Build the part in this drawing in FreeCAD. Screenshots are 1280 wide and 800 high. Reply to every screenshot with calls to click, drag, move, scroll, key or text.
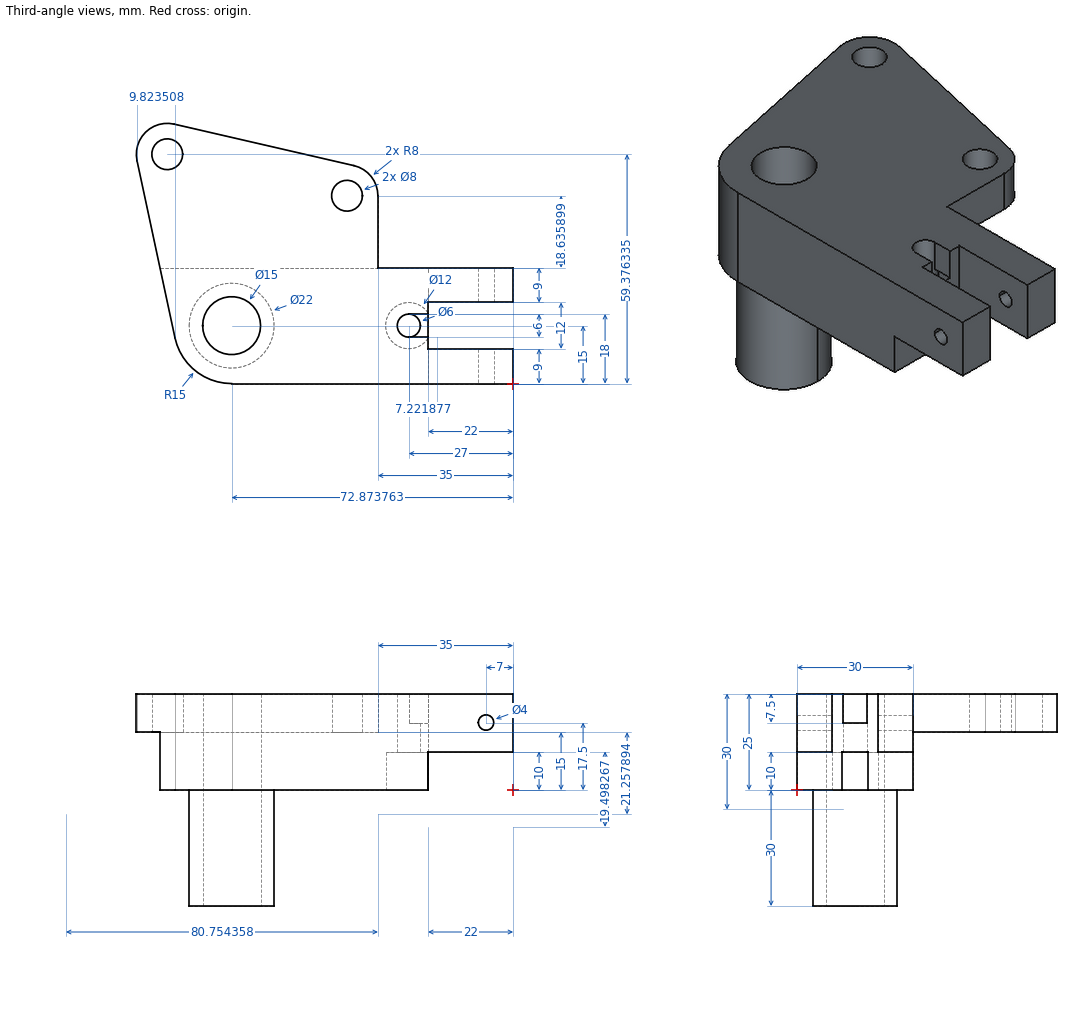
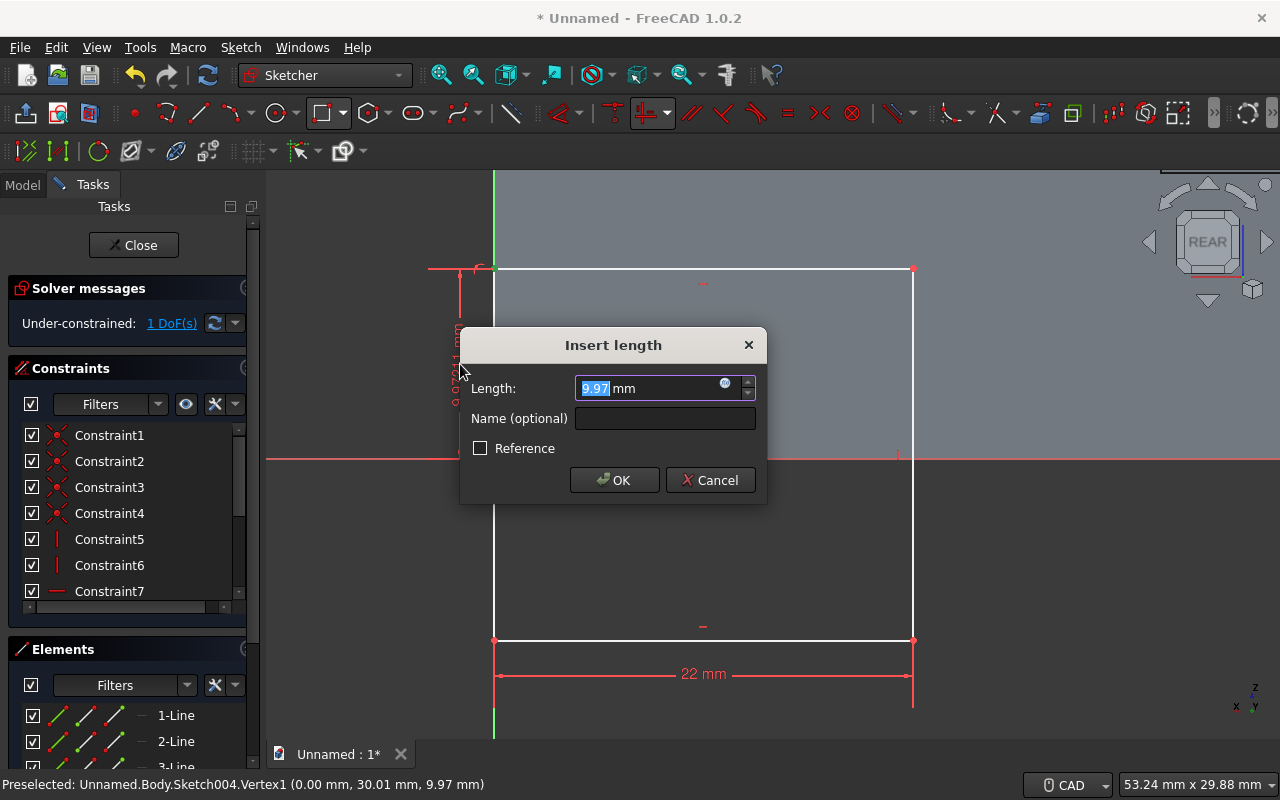
text(10)
key(Return)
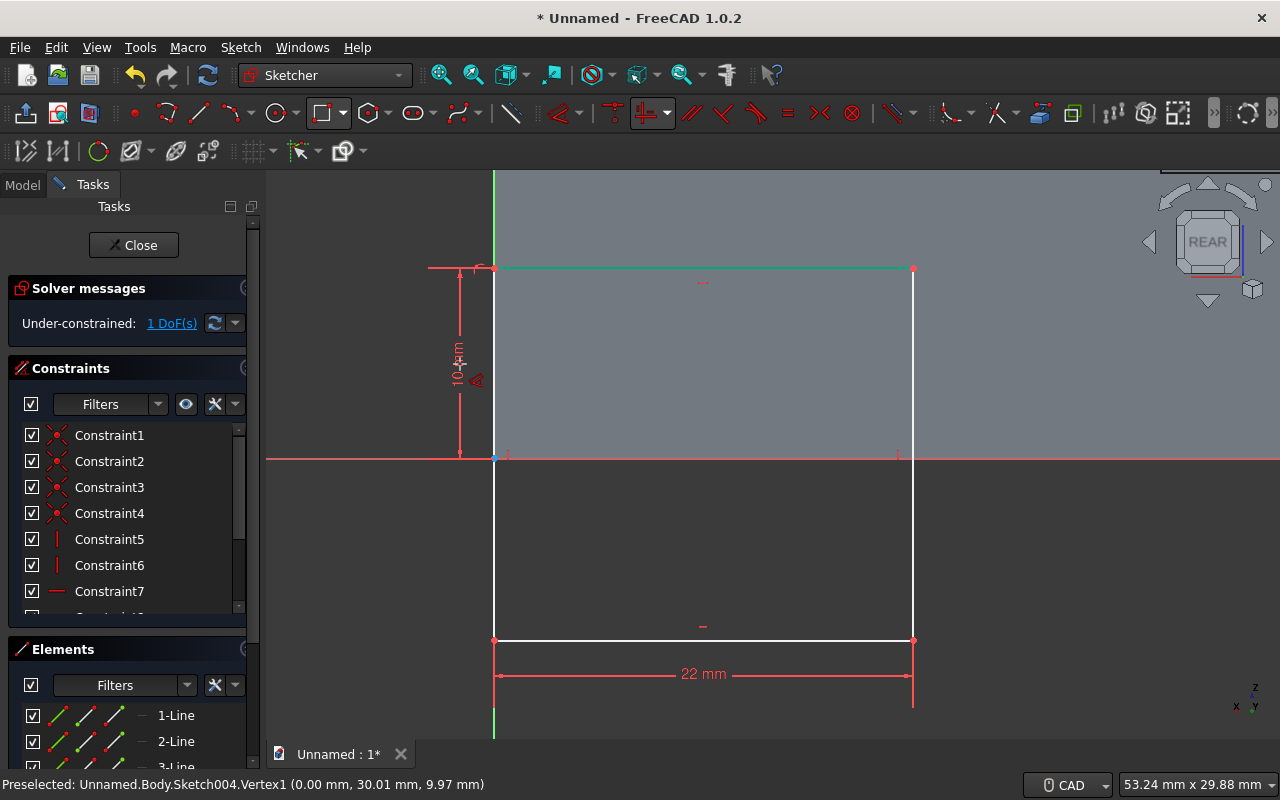
click(494, 380)
click(460, 540)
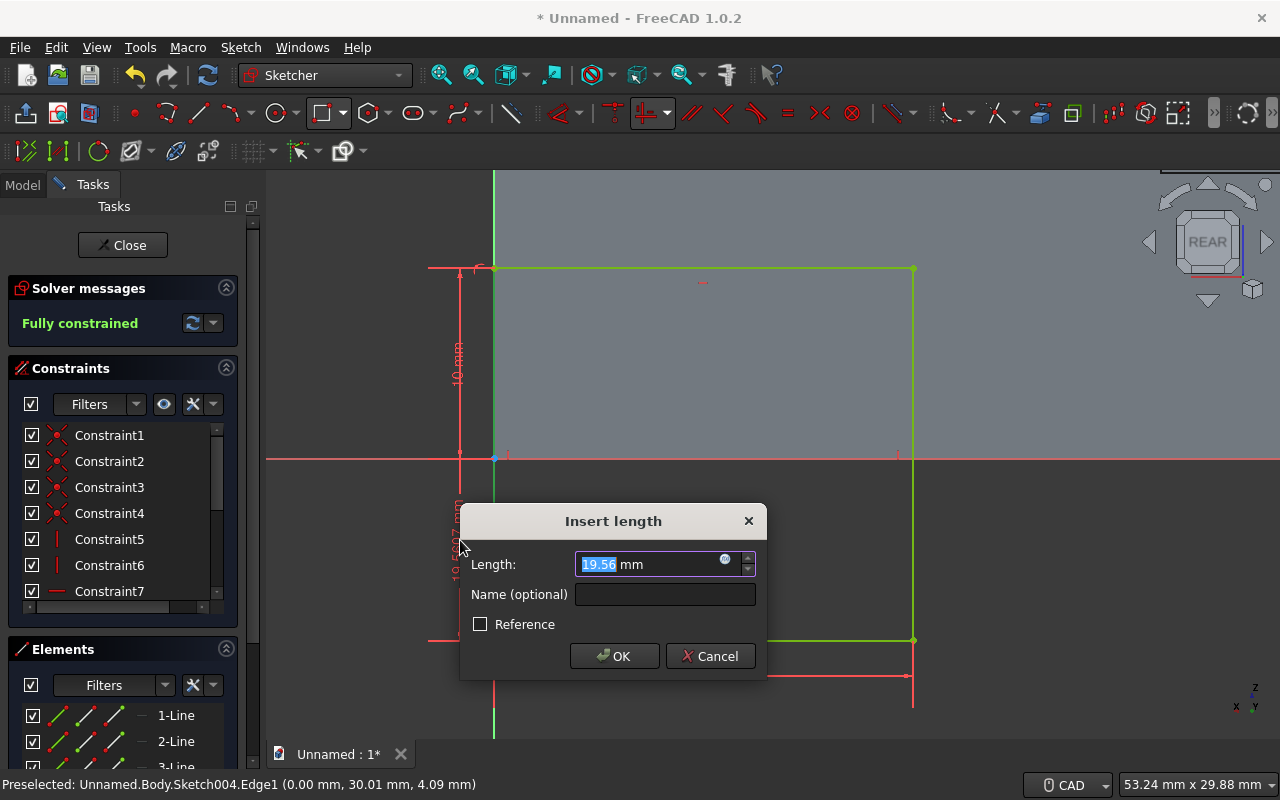
text(19.498267)
key(Return)
key(Escape)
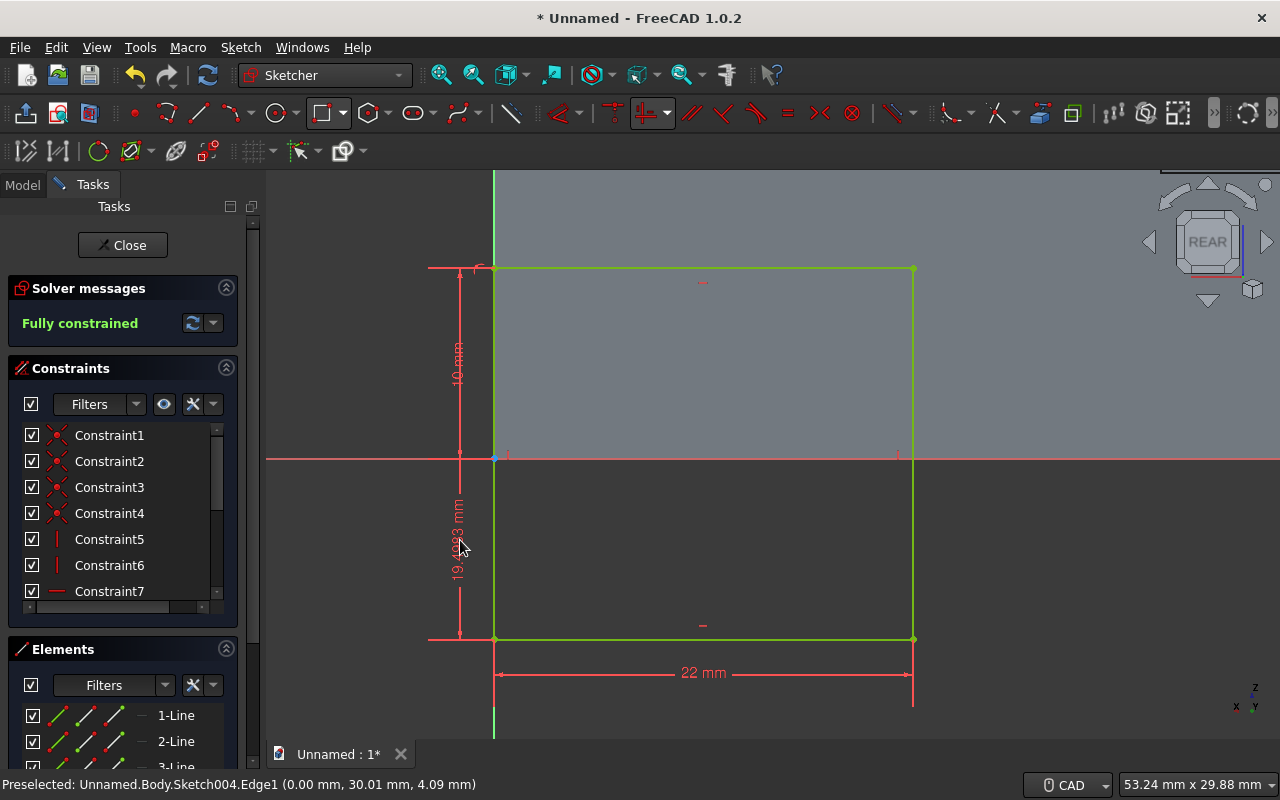
click(123, 245)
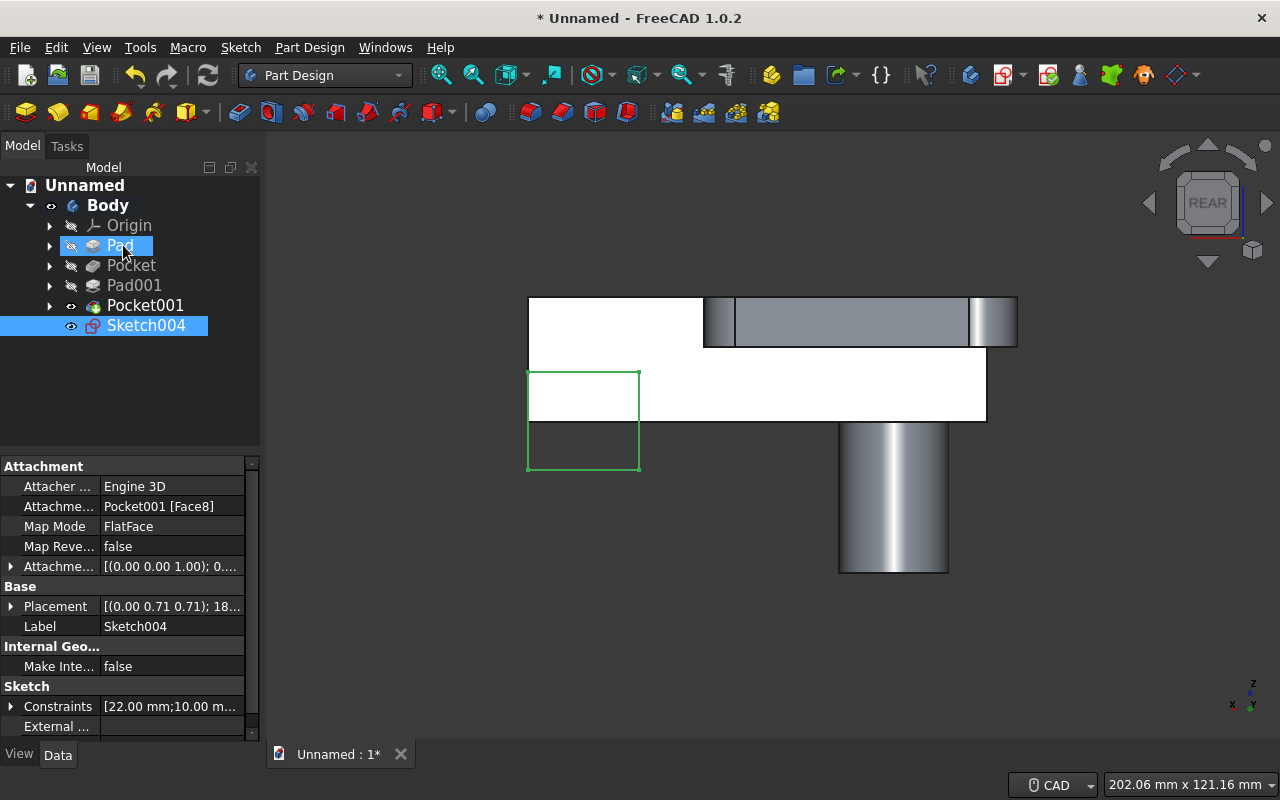
click(240, 112)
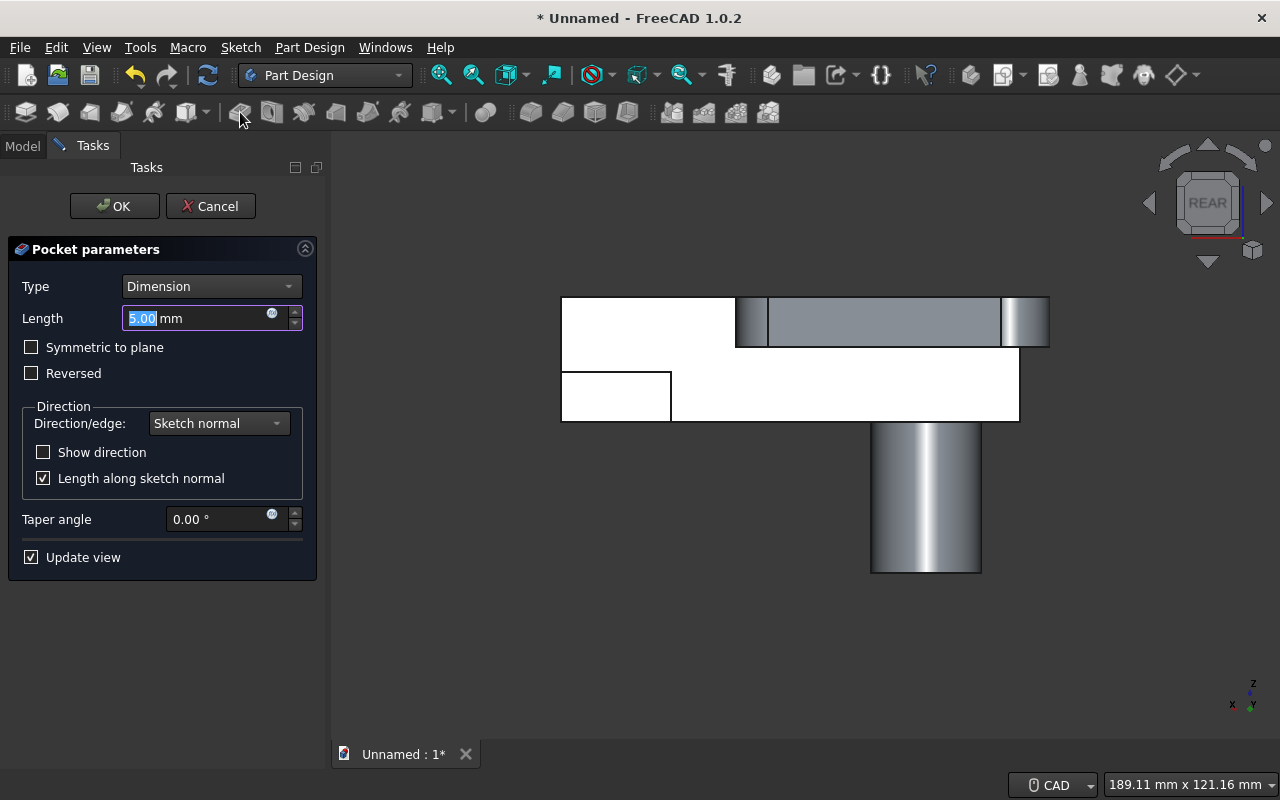
click(212, 286)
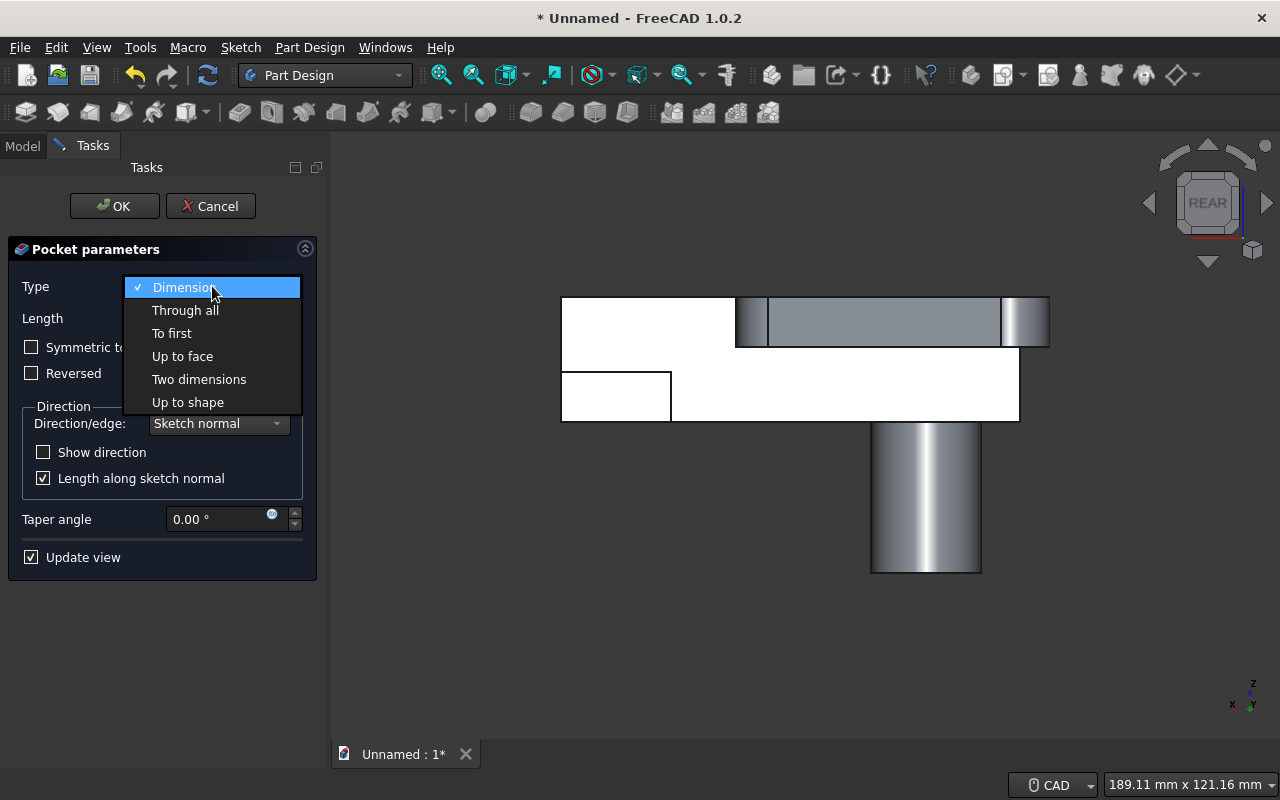
click(212, 310)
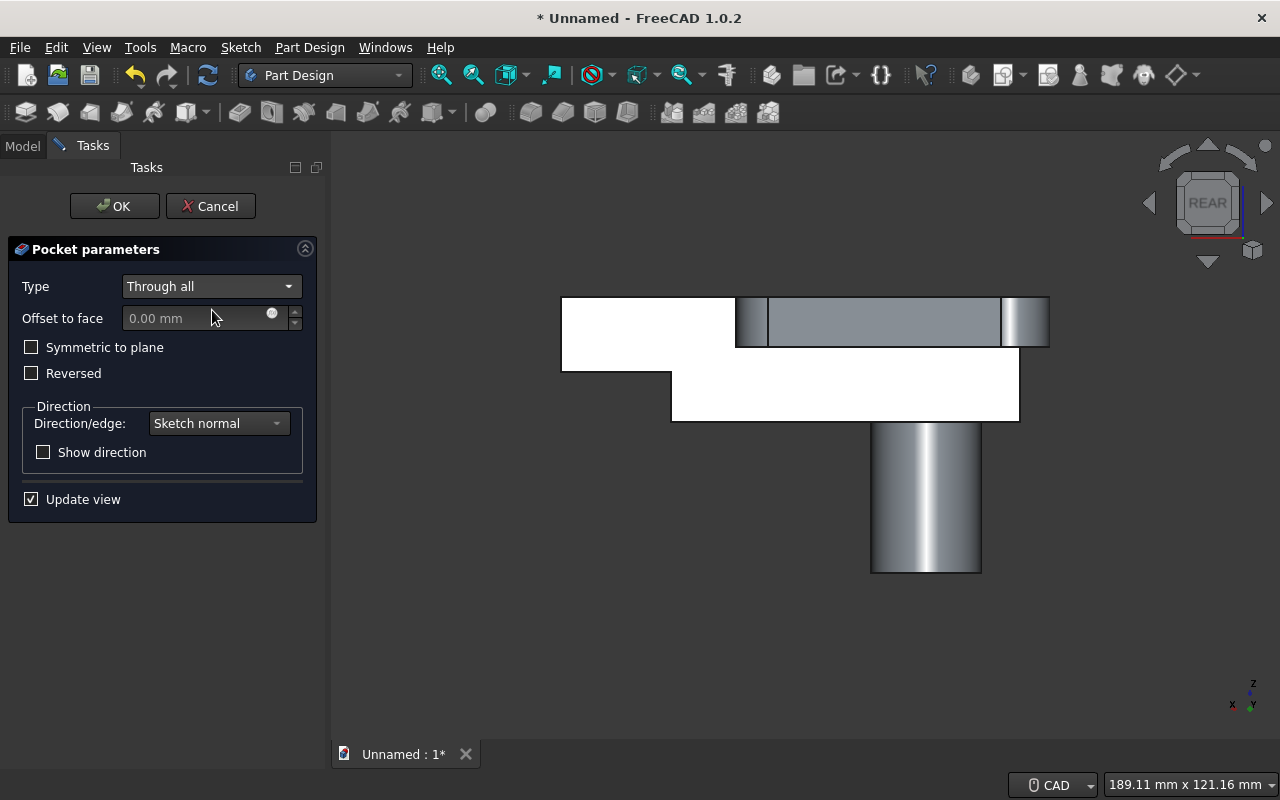
click(115, 206)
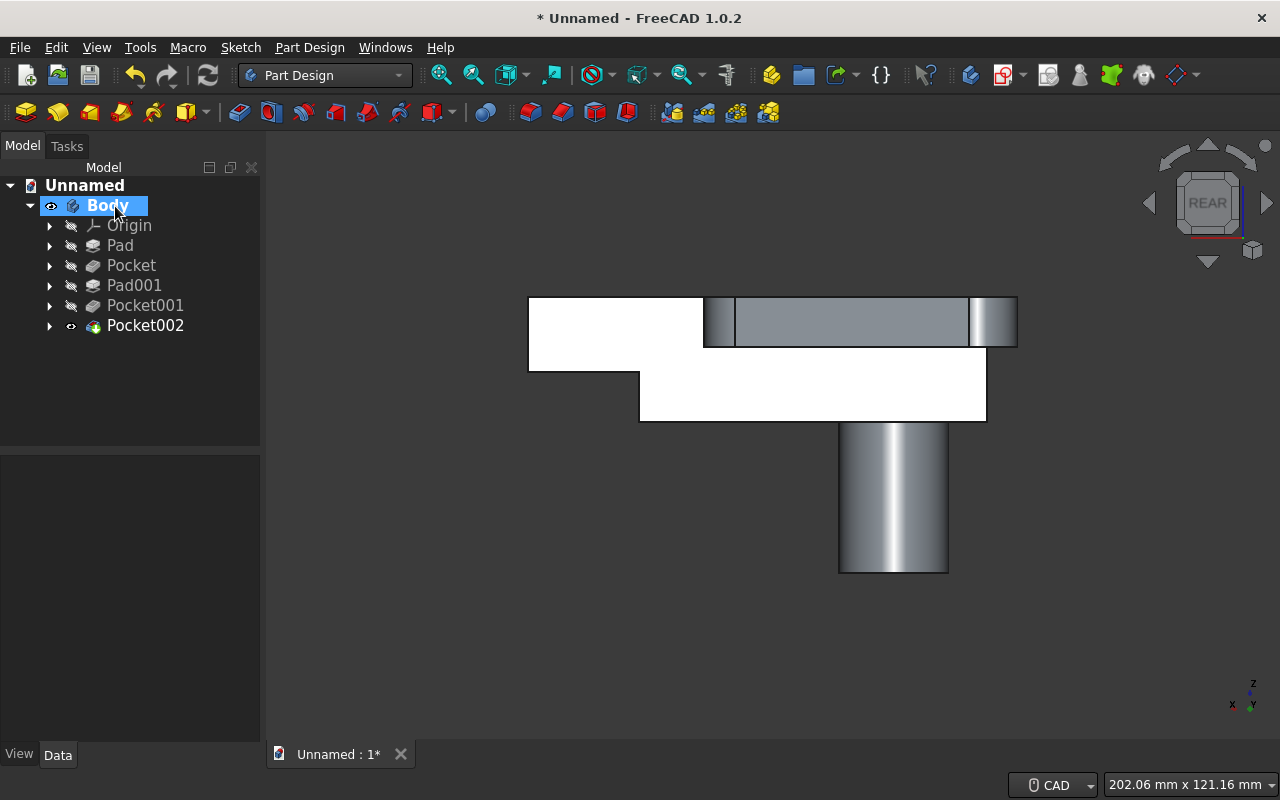
click(692, 377)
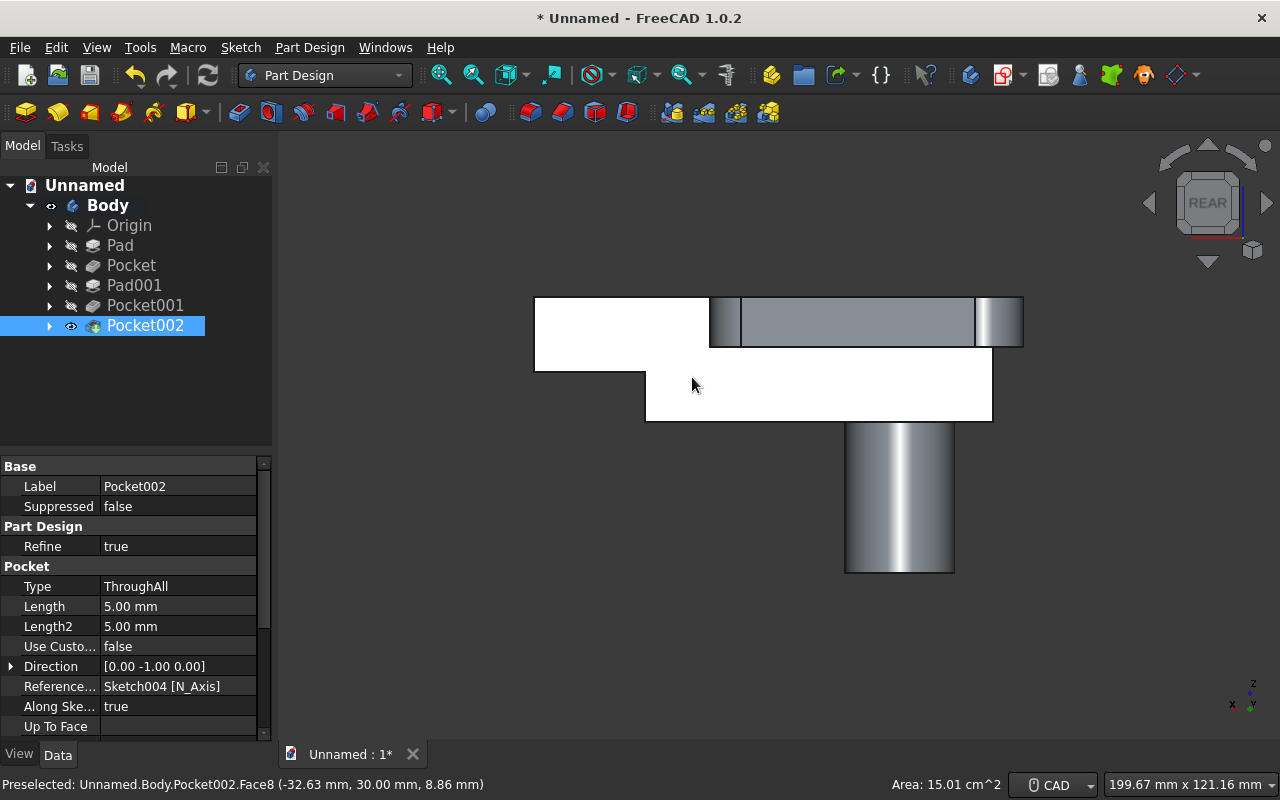
click(1004, 76)